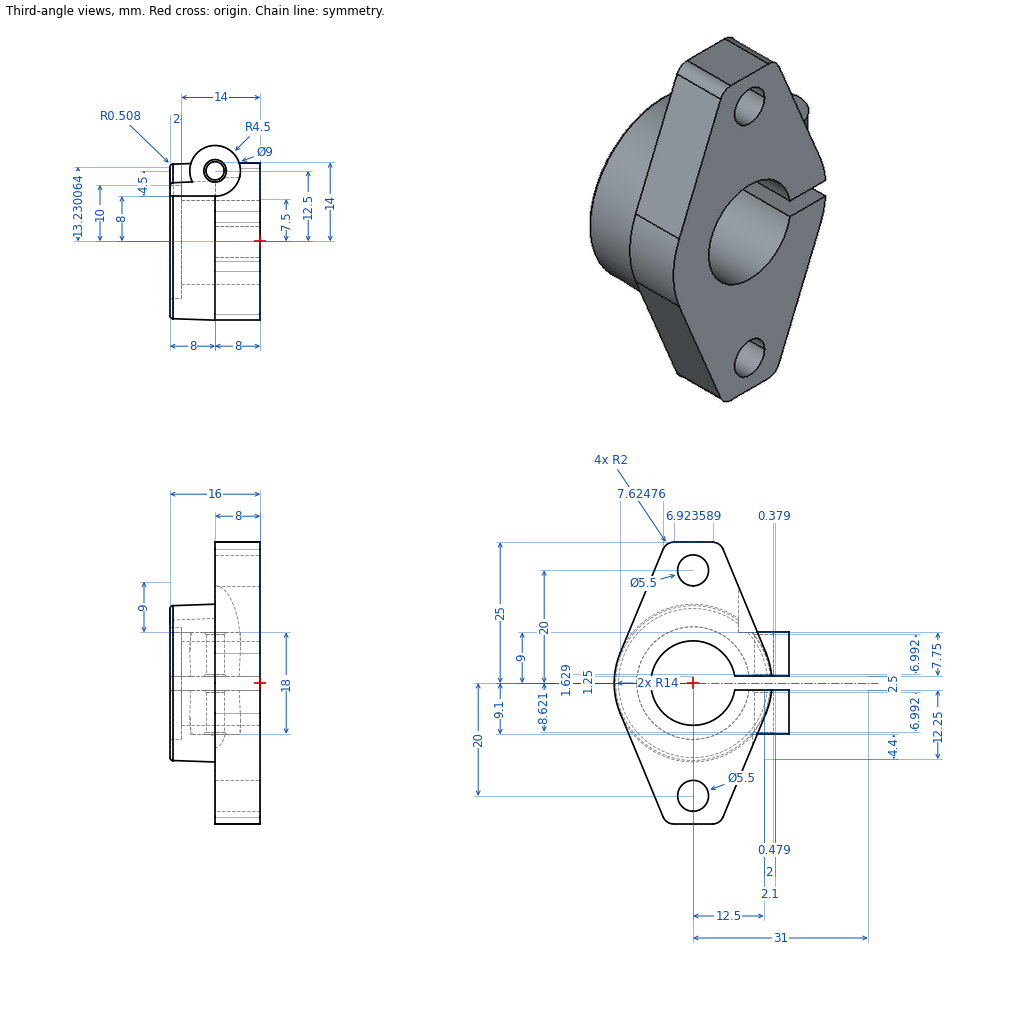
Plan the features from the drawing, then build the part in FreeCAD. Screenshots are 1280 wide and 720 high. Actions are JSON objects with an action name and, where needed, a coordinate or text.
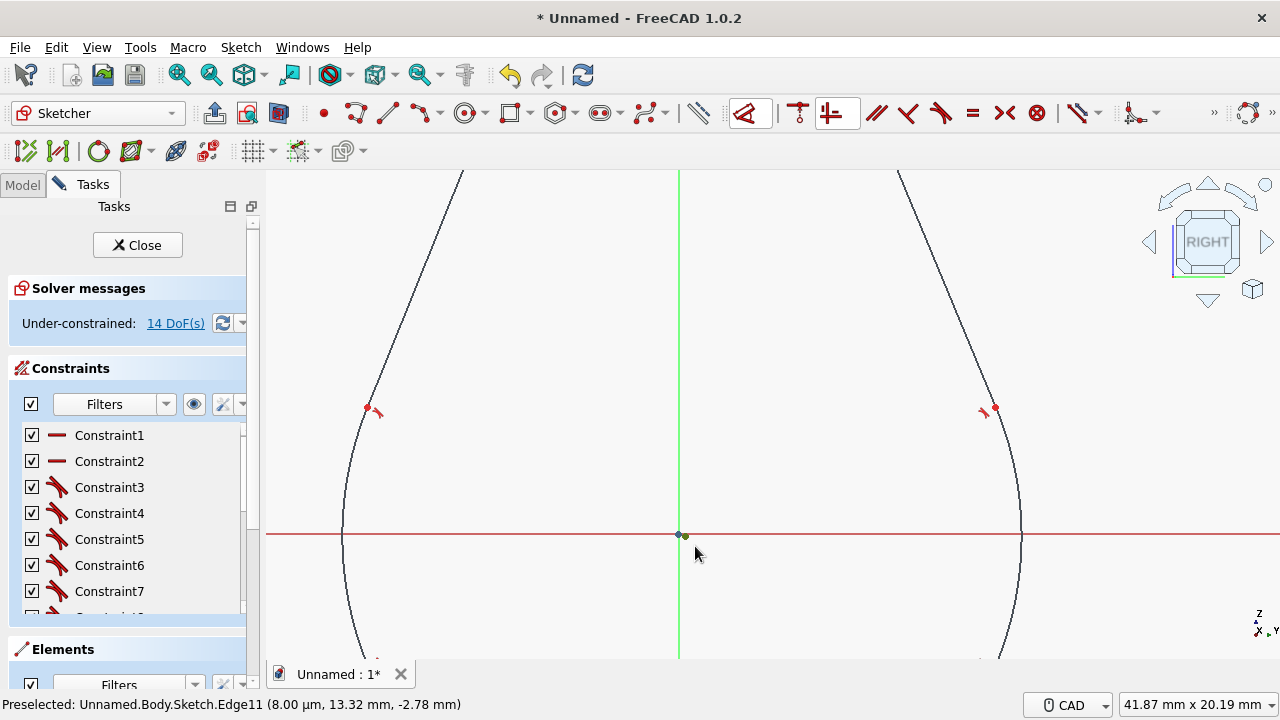
{"action": "left_click", "coordinate": [798, 114]}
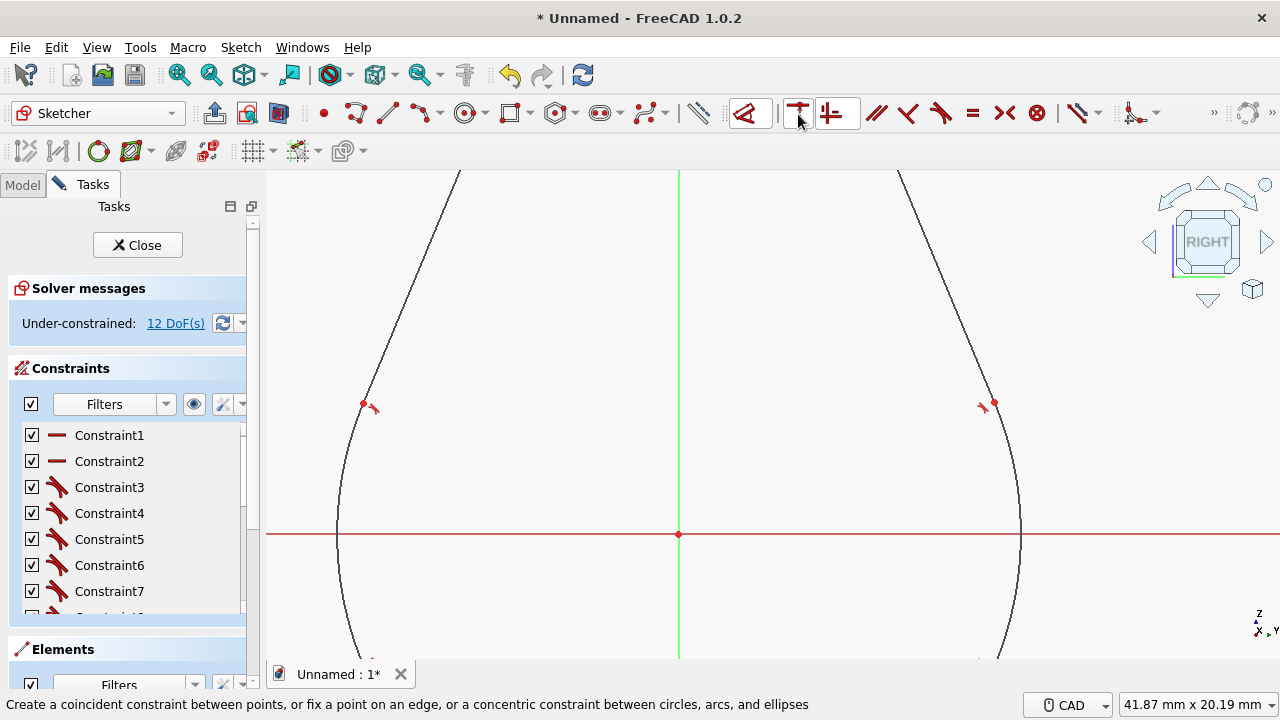
{"action": "scroll", "coordinate": [713, 375], "scroll_direction": "down", "scroll_amount": 7}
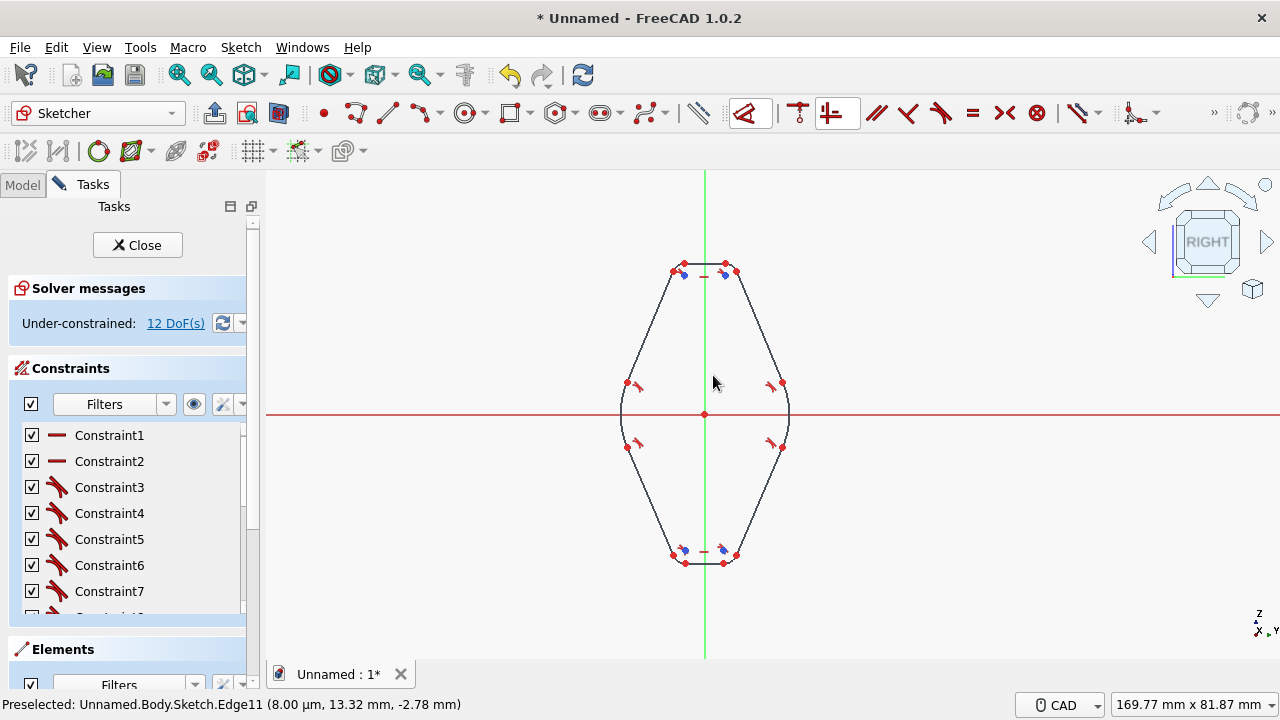
{"action": "scroll", "coordinate": [680, 265], "scroll_direction": "up", "scroll_amount": 7}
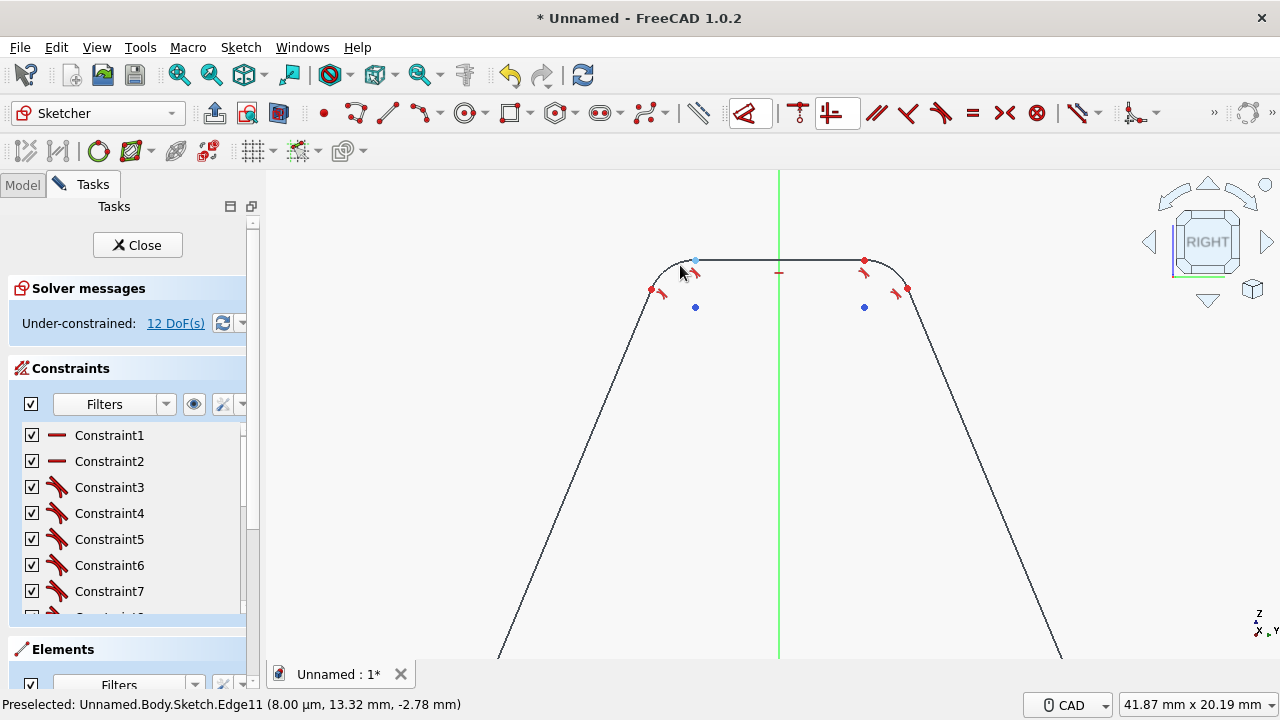
{"action": "left_click", "coordinate": [679, 263]}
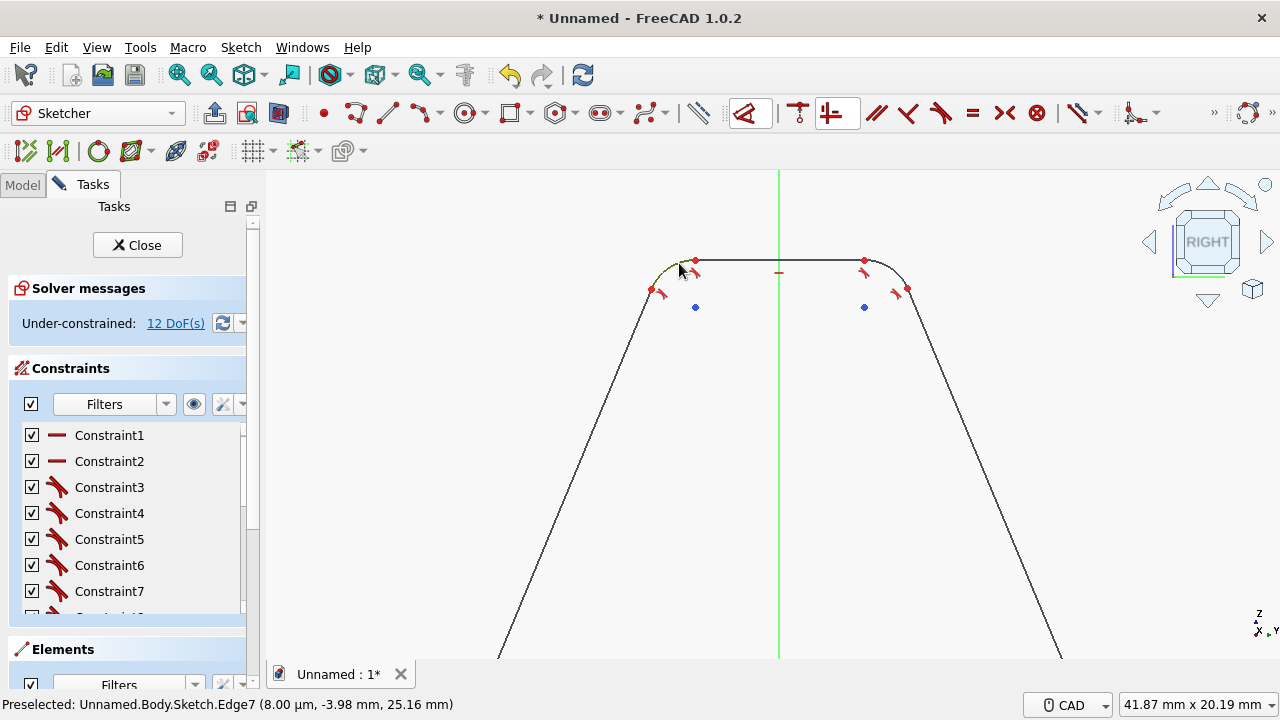
{"action": "scroll", "coordinate": [680, 265], "scroll_direction": "down", "scroll_amount": 7}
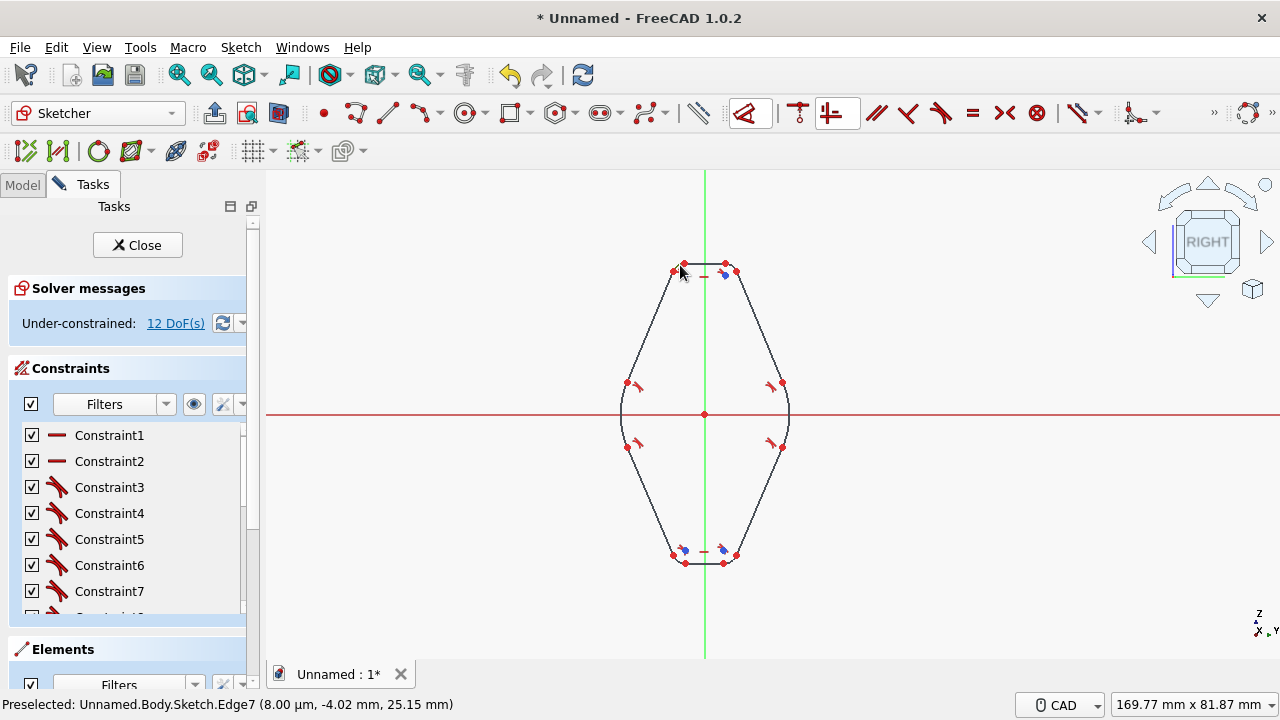
{"action": "scroll", "coordinate": [676, 560], "scroll_direction": "up", "scroll_amount": 6}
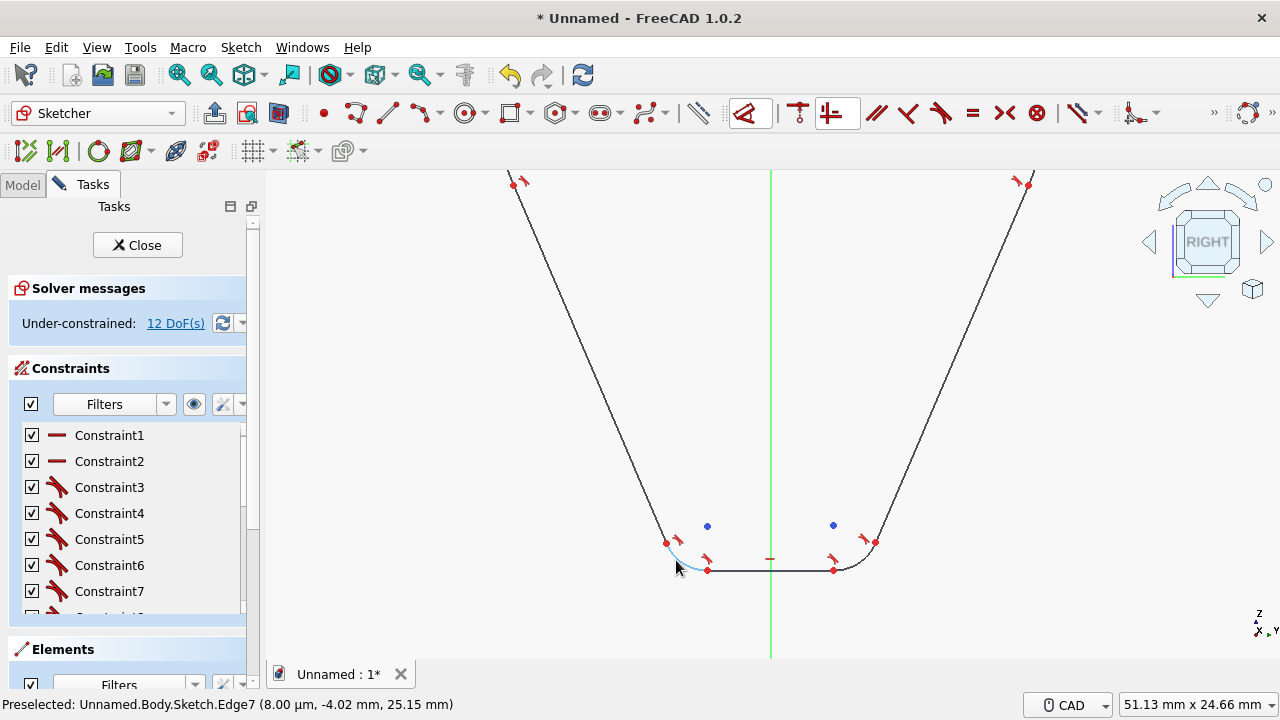
{"action": "left_click", "coordinate": [675, 557]}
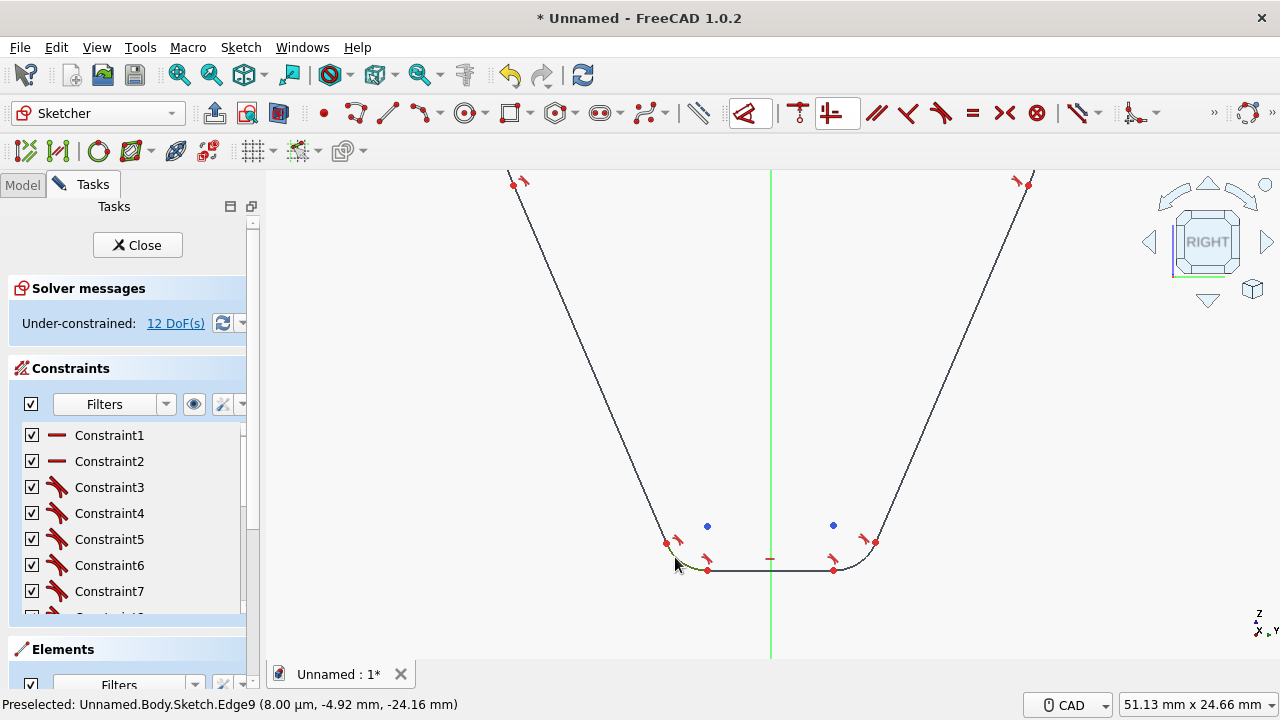
{"action": "left_click", "coordinate": [849, 568]}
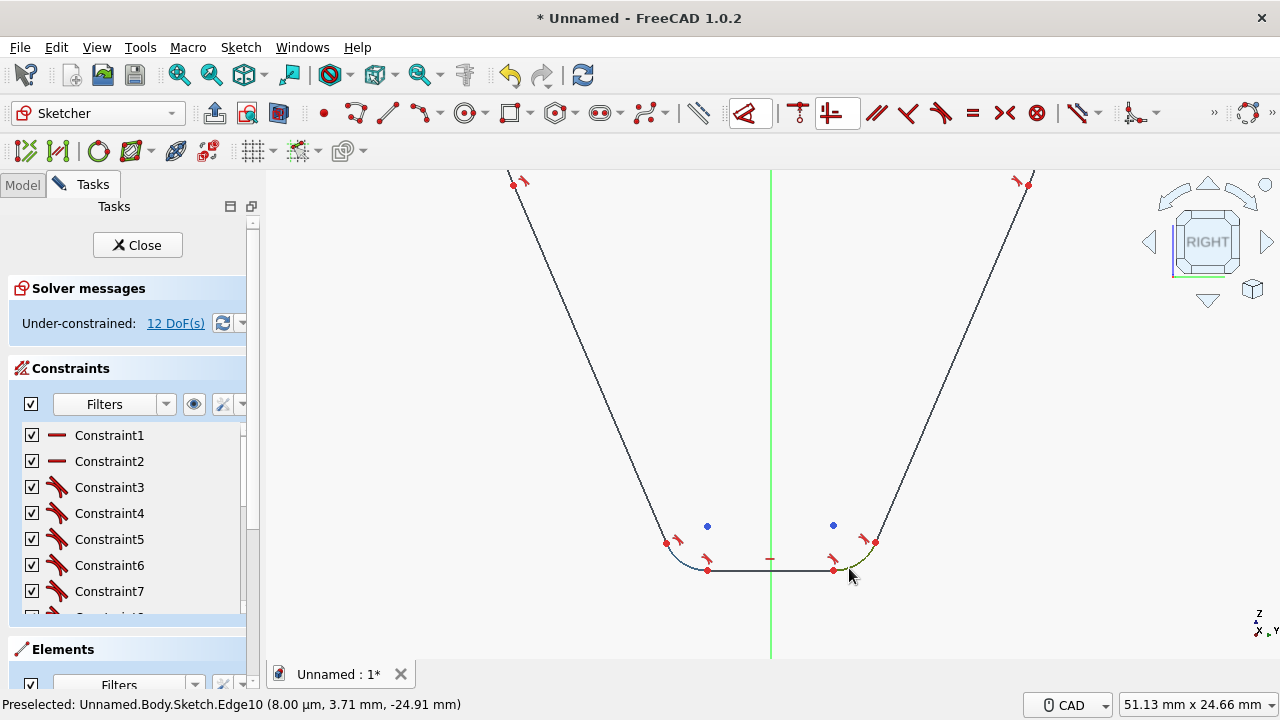
{"action": "scroll", "coordinate": [676, 561], "scroll_direction": "down", "scroll_amount": 6}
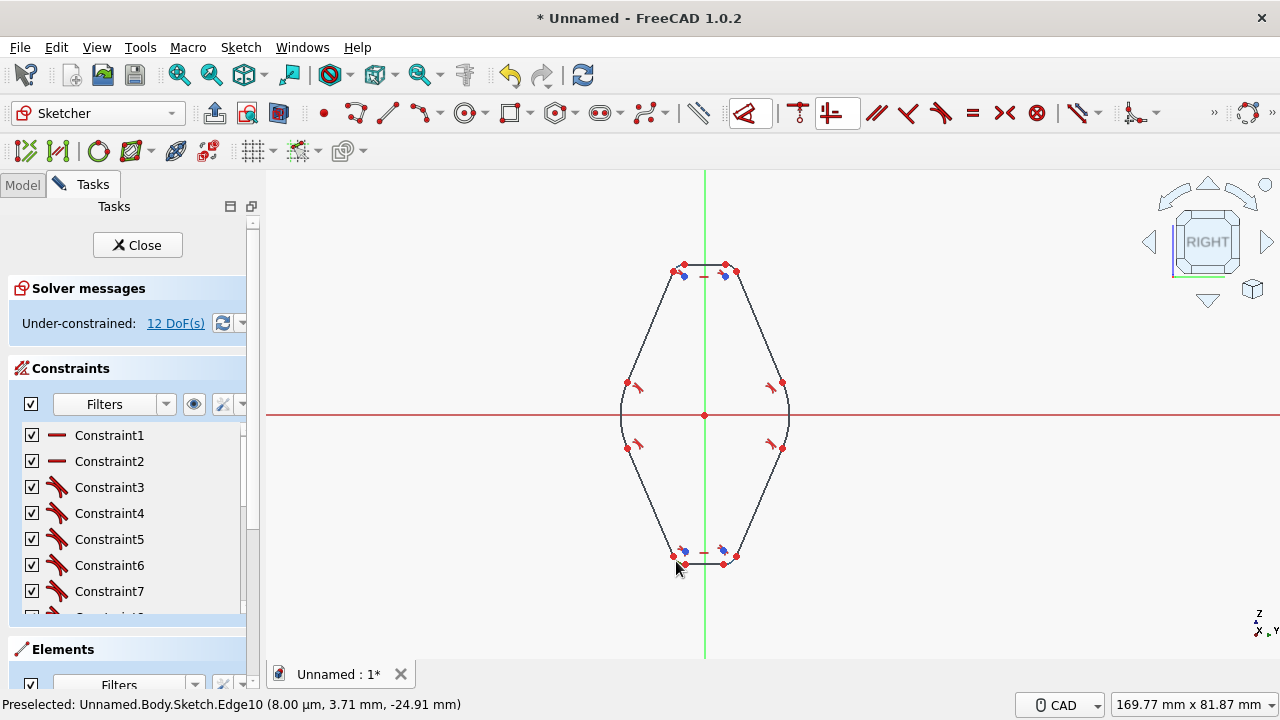
{"action": "scroll", "coordinate": [734, 268], "scroll_direction": "up", "scroll_amount": 7}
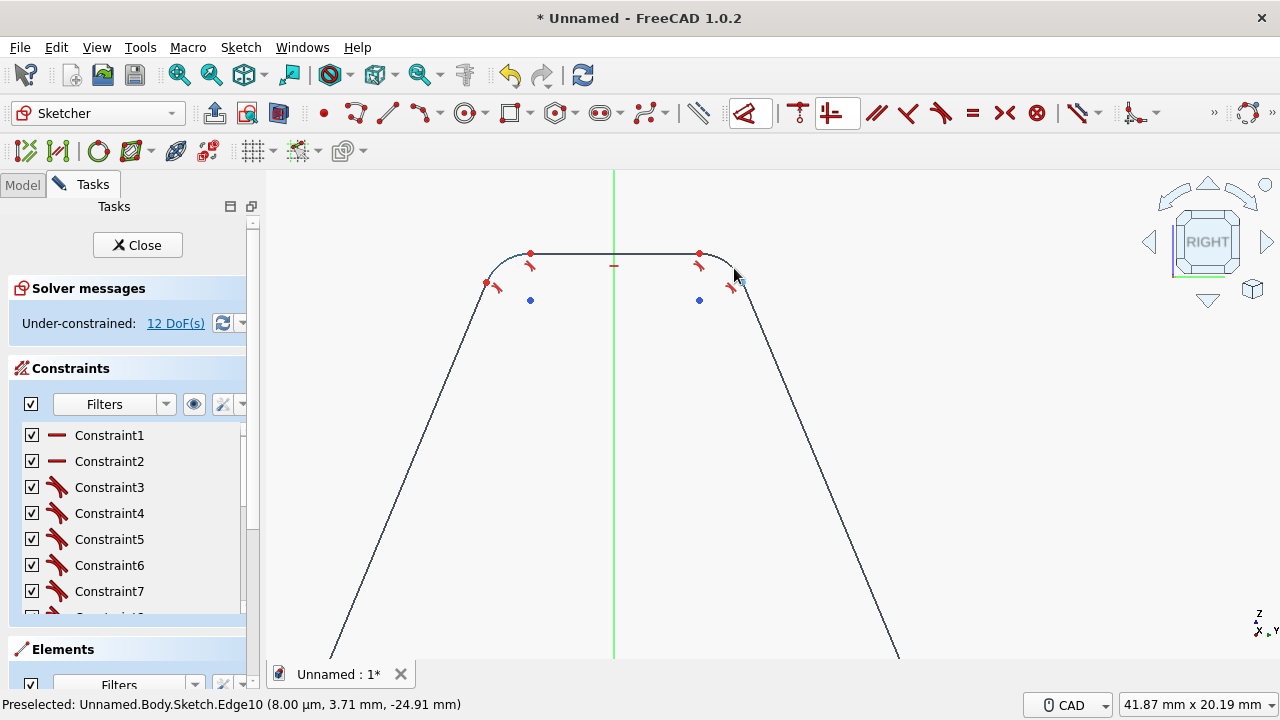
{"action": "left_click", "coordinate": [734, 269]}